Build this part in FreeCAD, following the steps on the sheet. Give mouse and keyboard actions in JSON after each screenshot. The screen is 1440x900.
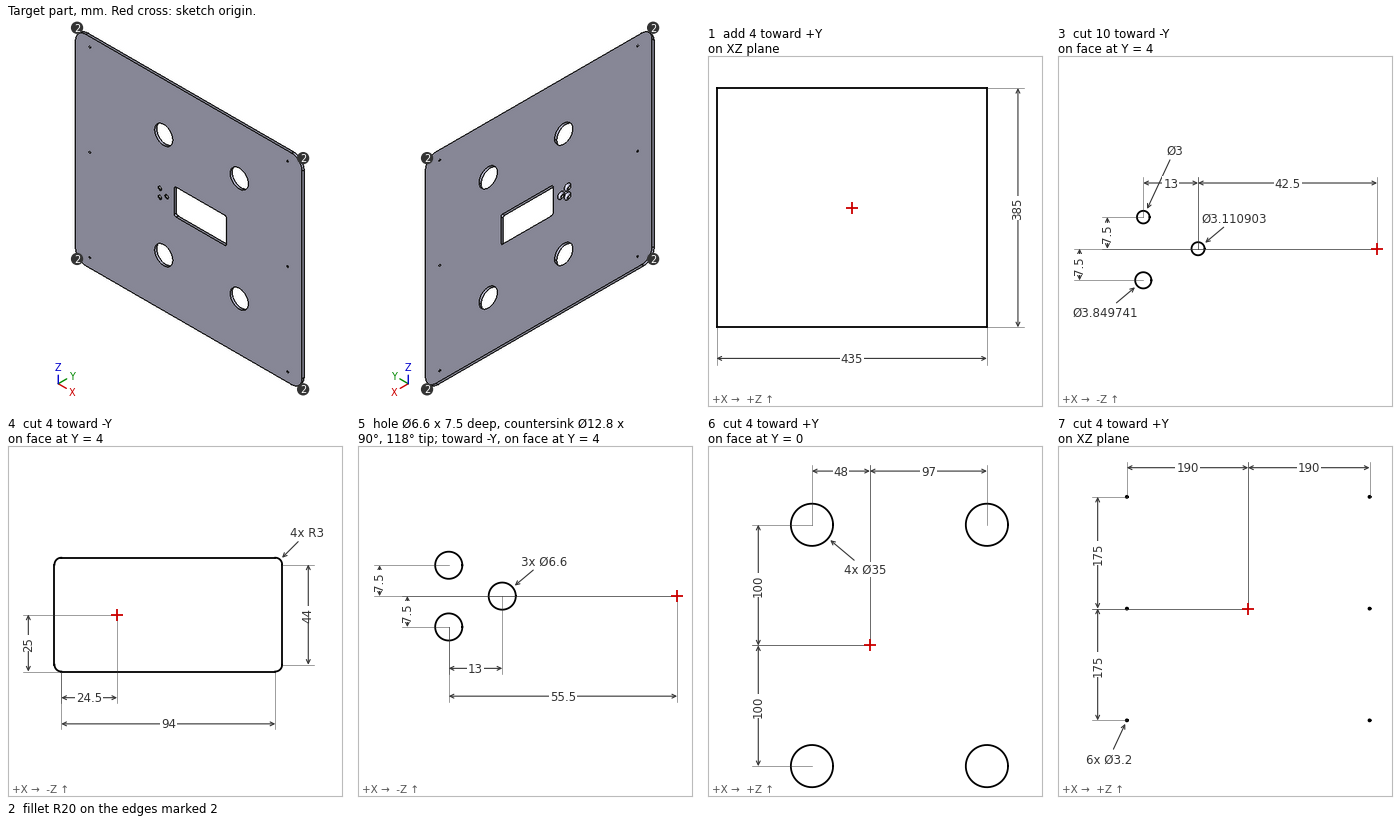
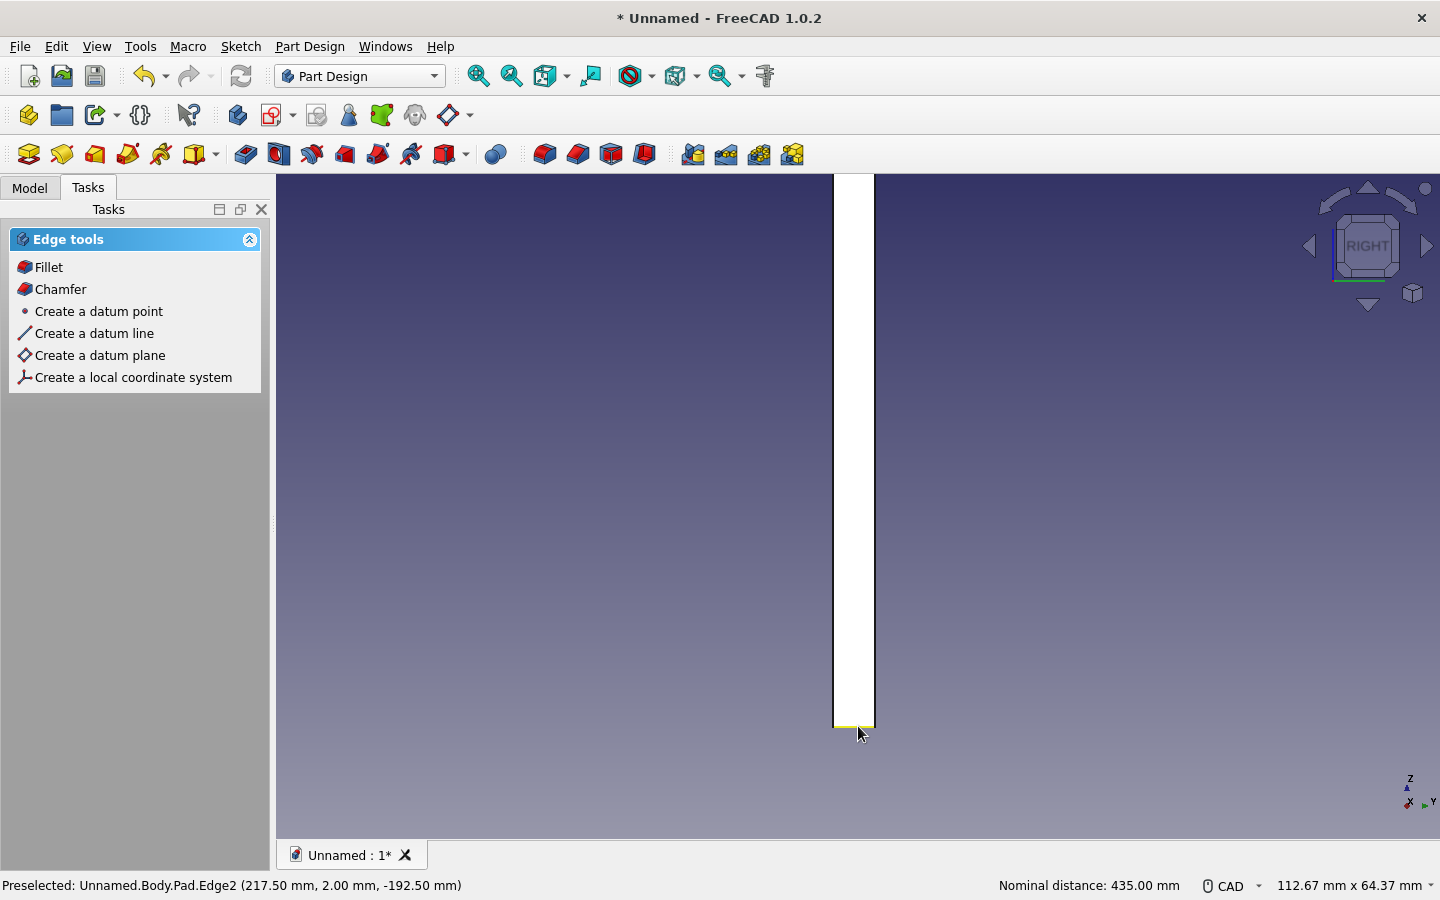
{"action": "left_click", "coordinate": [854, 726], "text": "ctrl"}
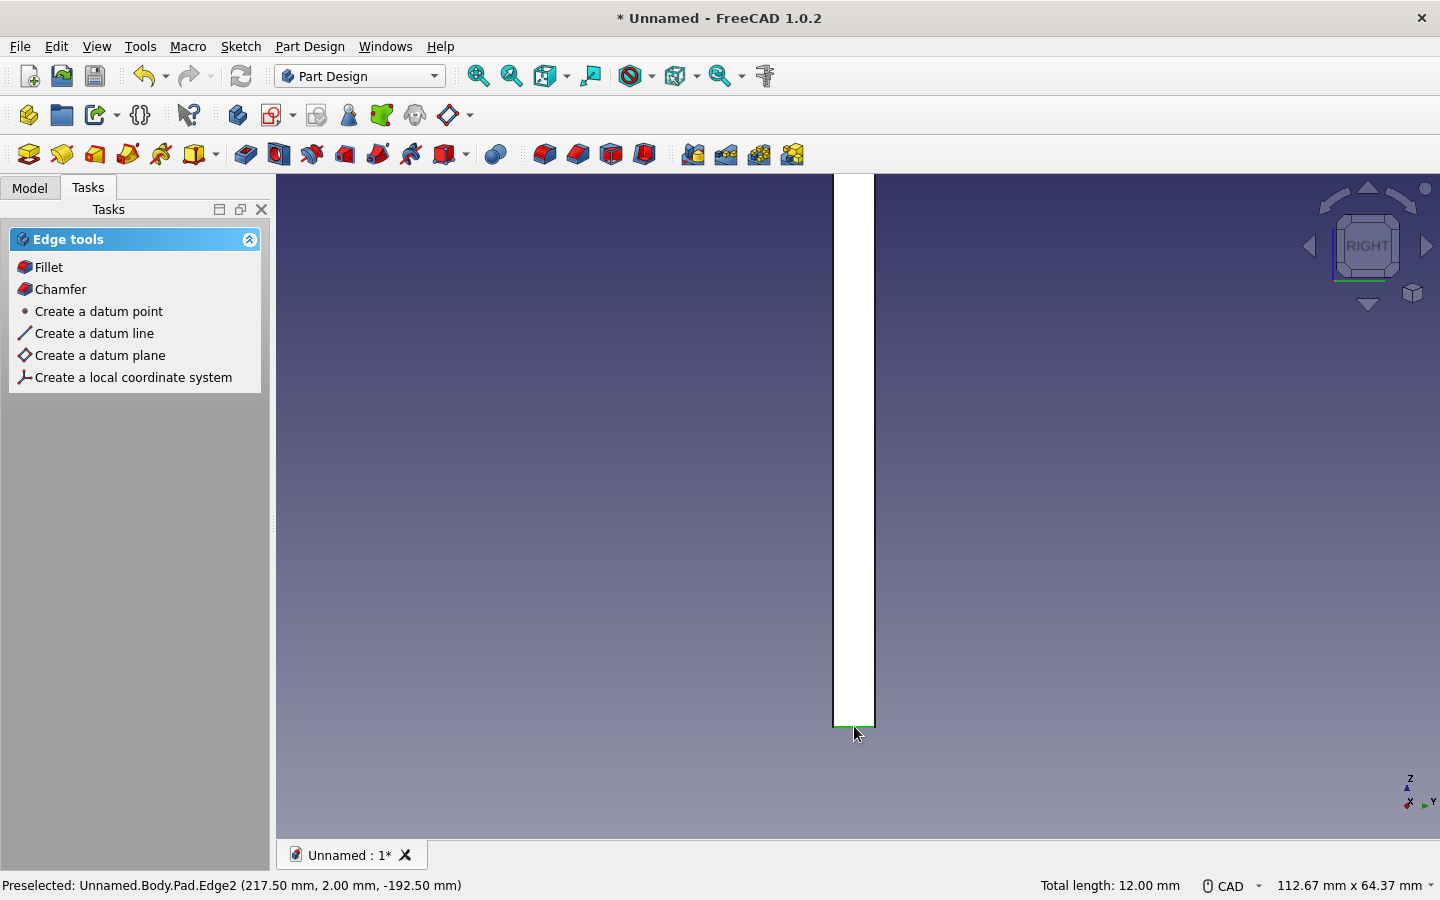
{"action": "left_click", "coordinate": [479, 76]}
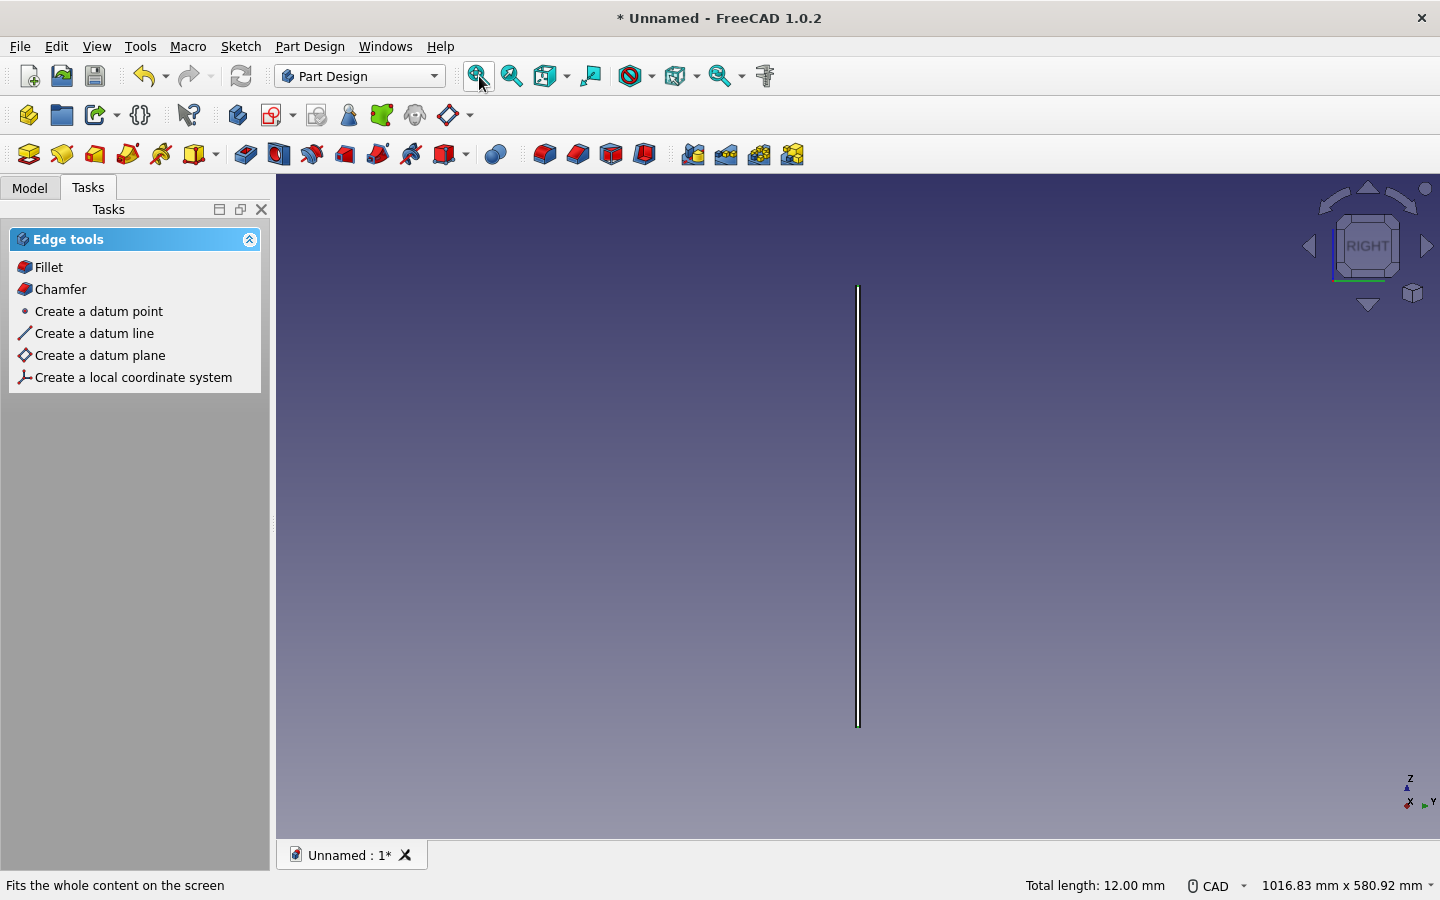
{"action": "key", "text": "5"}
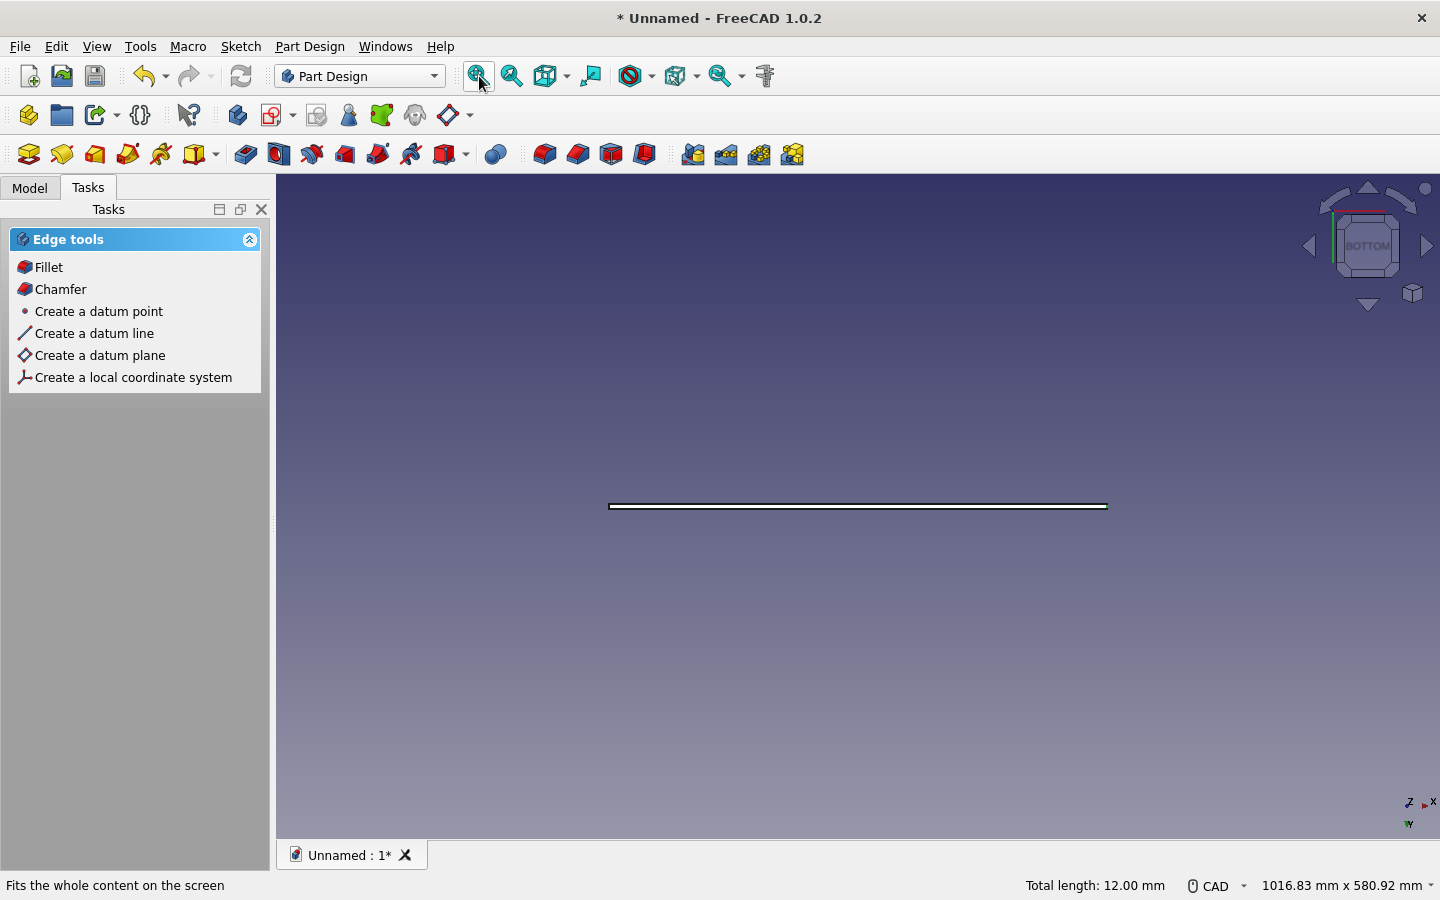
{"action": "left_click", "coordinate": [479, 76]}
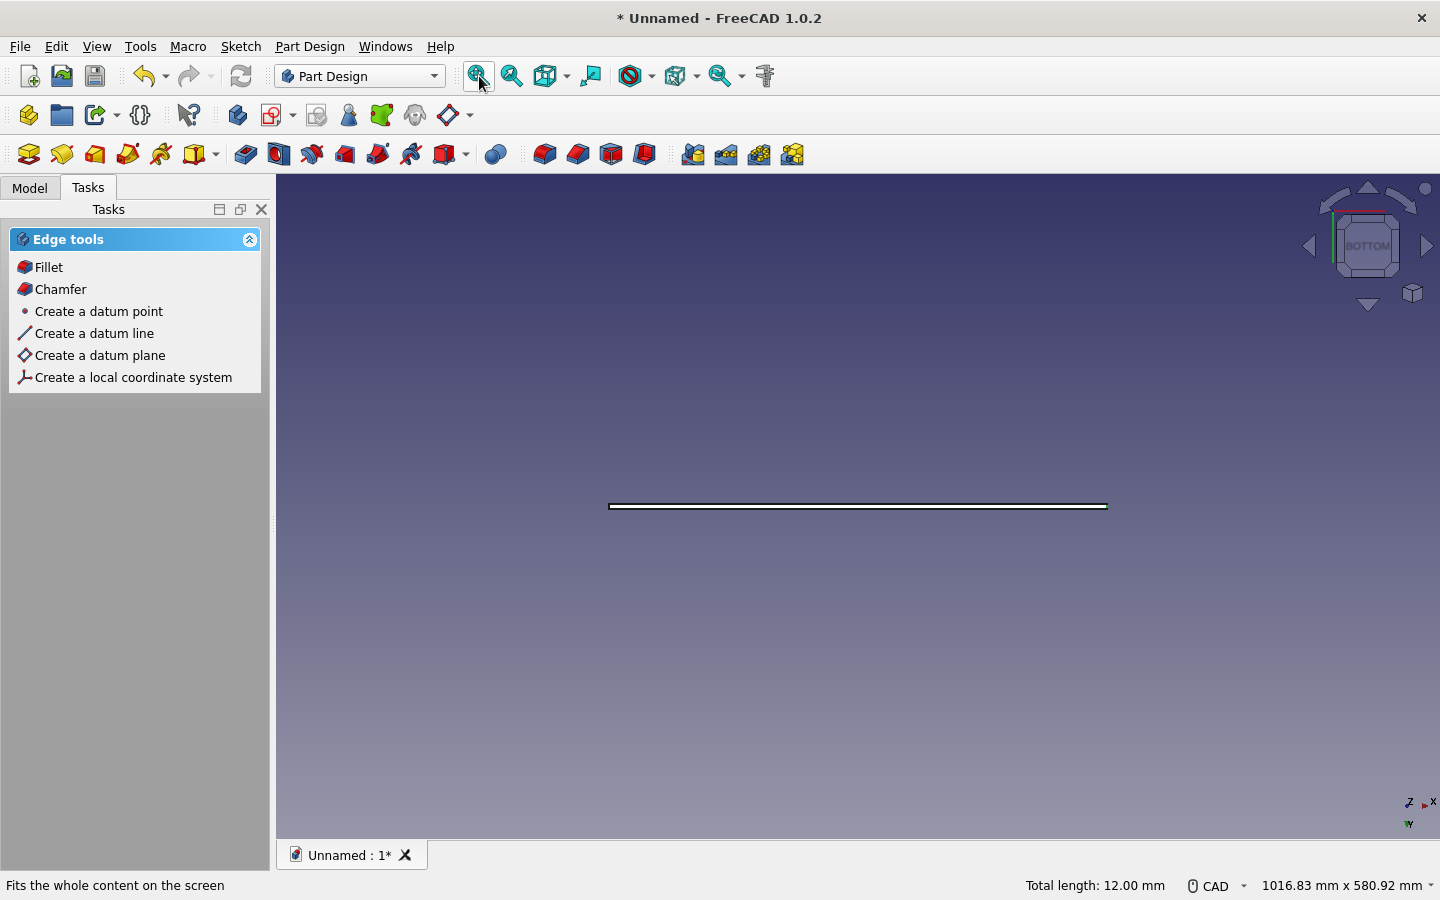
{"action": "scroll", "coordinate": [609, 505], "scroll_direction": "up", "scroll_amount": 11}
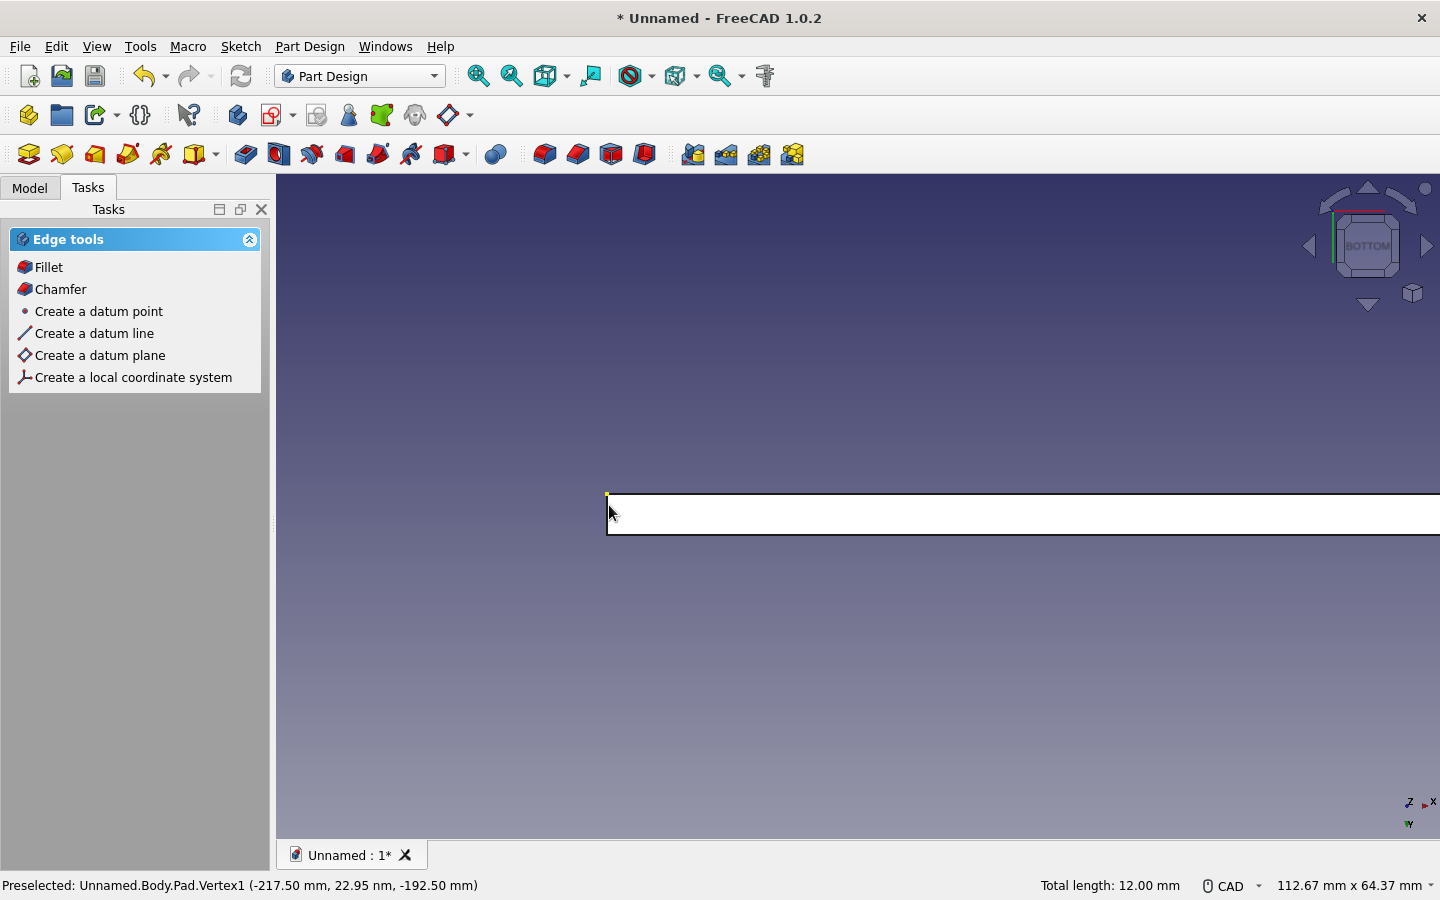
{"action": "left_click", "coordinate": [607, 514], "text": "ctrl"}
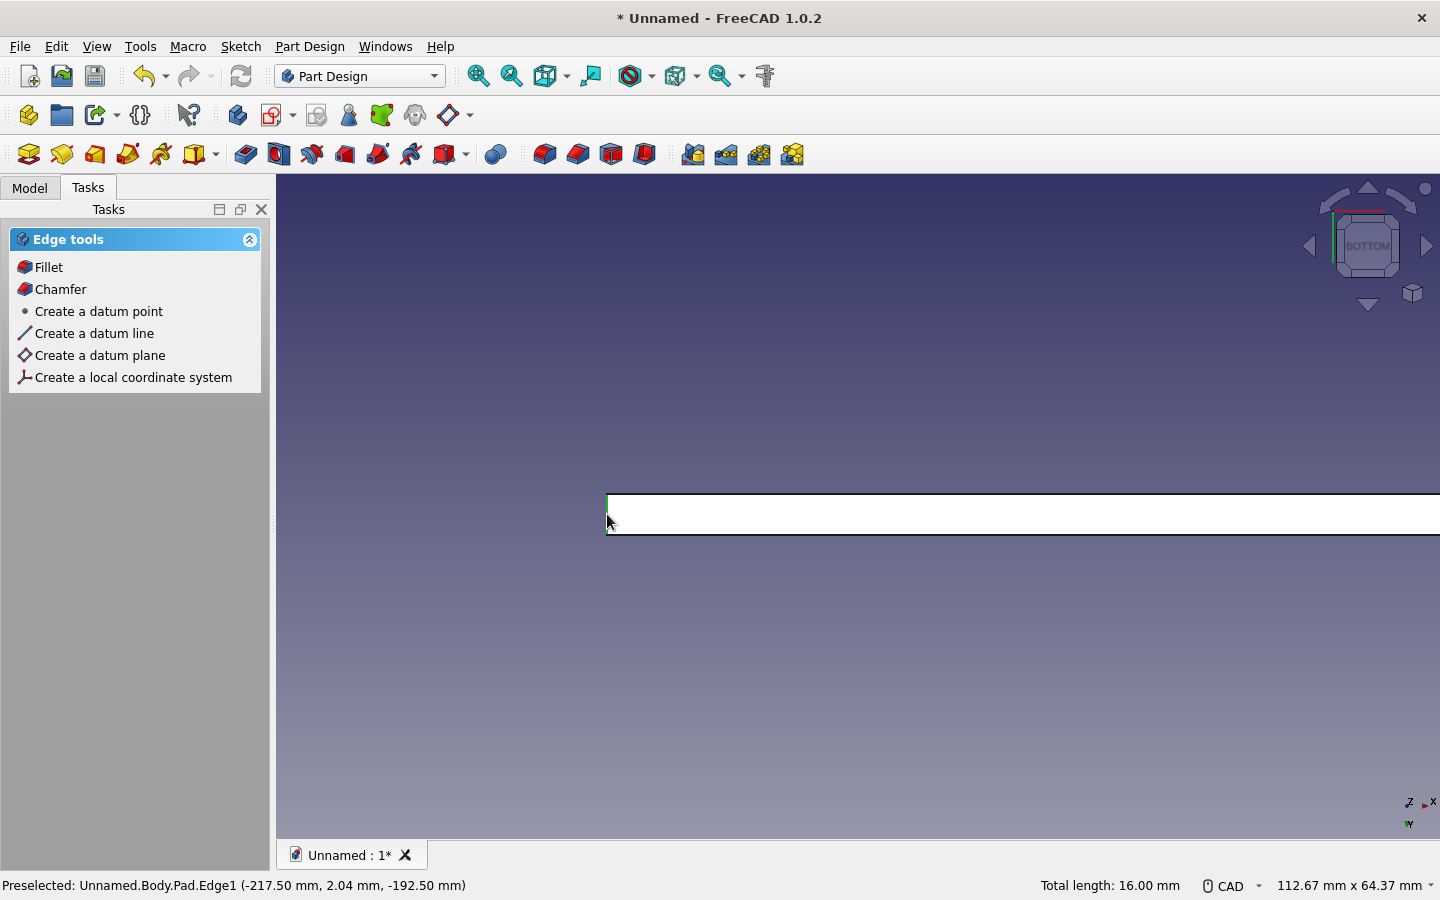
{"action": "left_click", "coordinate": [545, 154]}